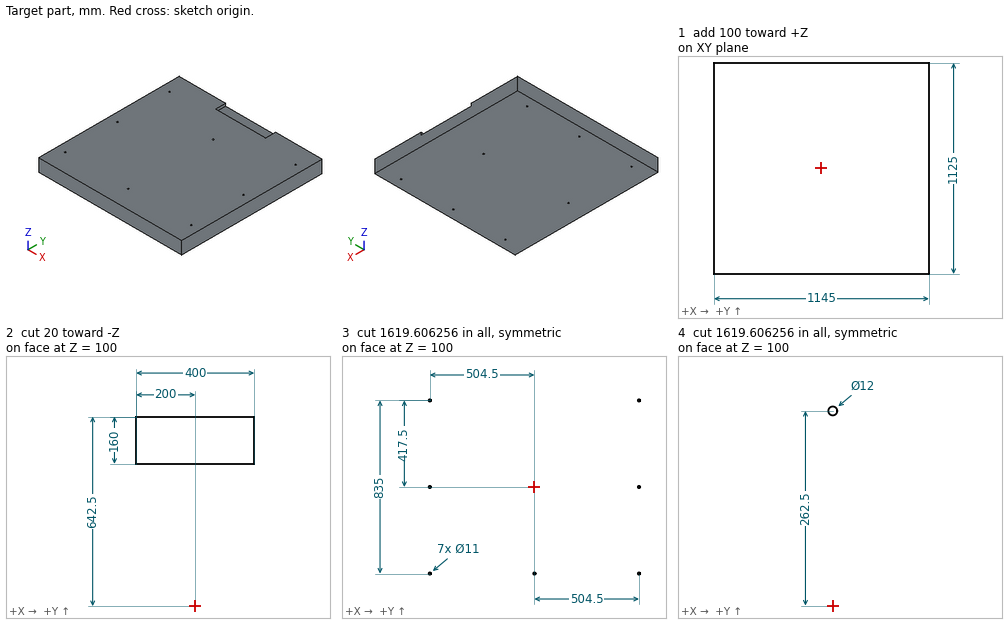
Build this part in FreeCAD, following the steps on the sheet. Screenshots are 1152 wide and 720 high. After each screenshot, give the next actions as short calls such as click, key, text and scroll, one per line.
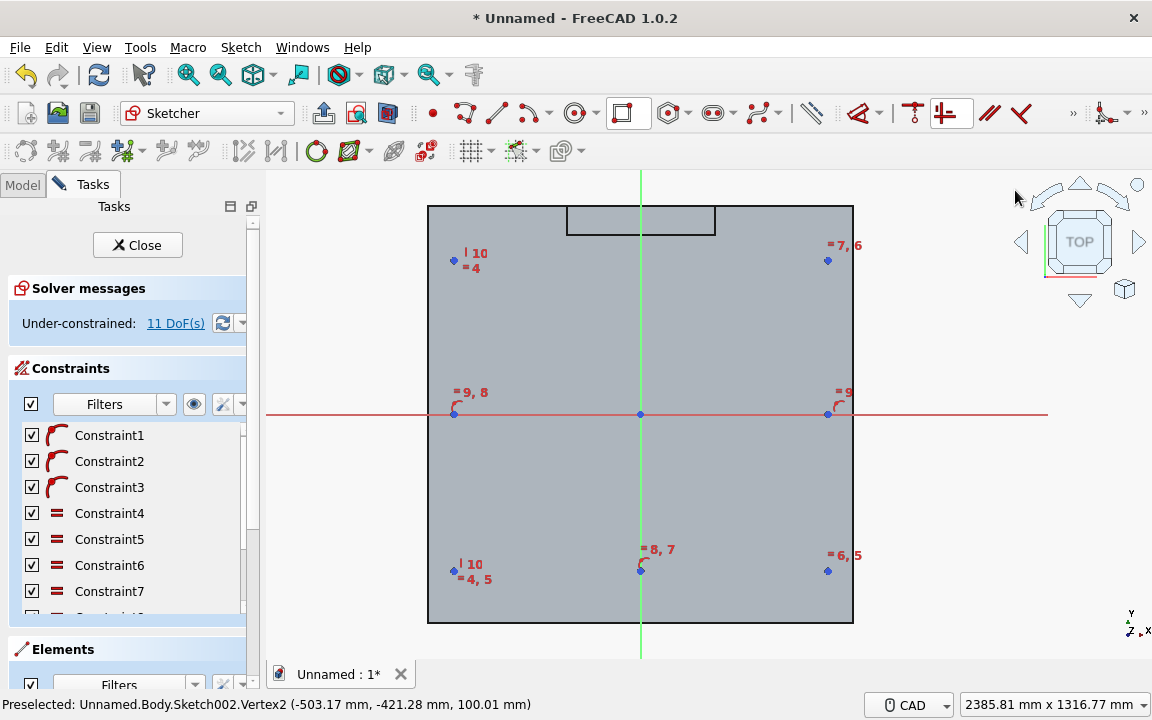
click(454, 571)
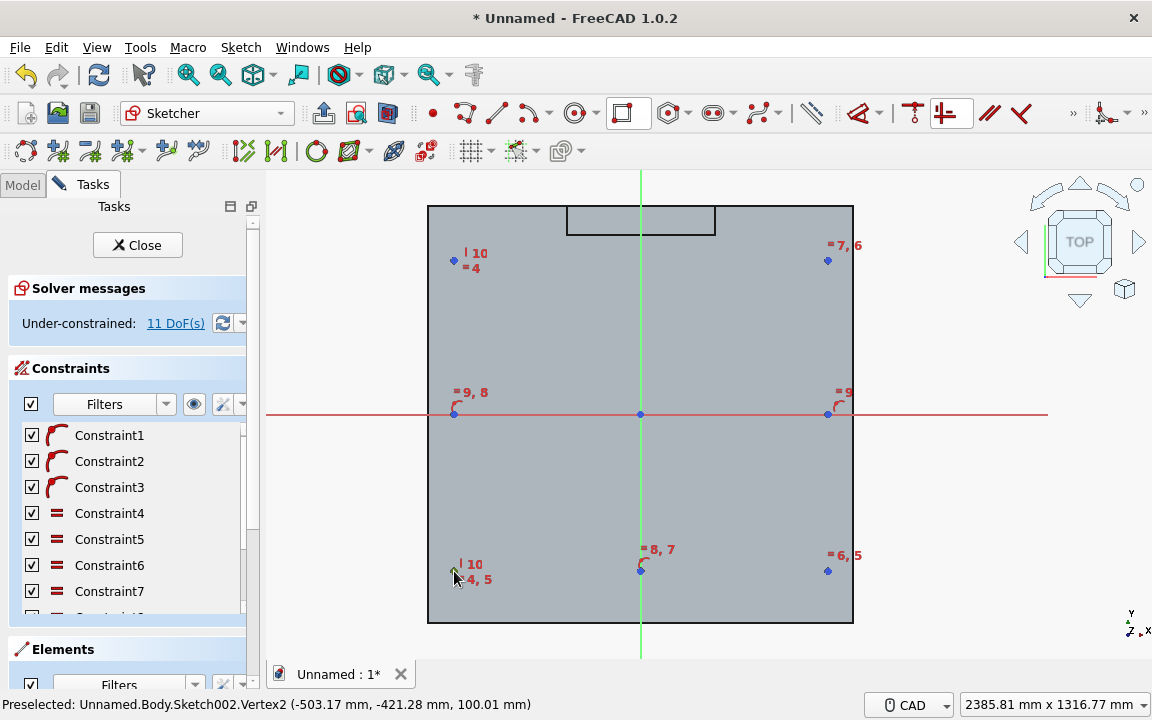
click(828, 571)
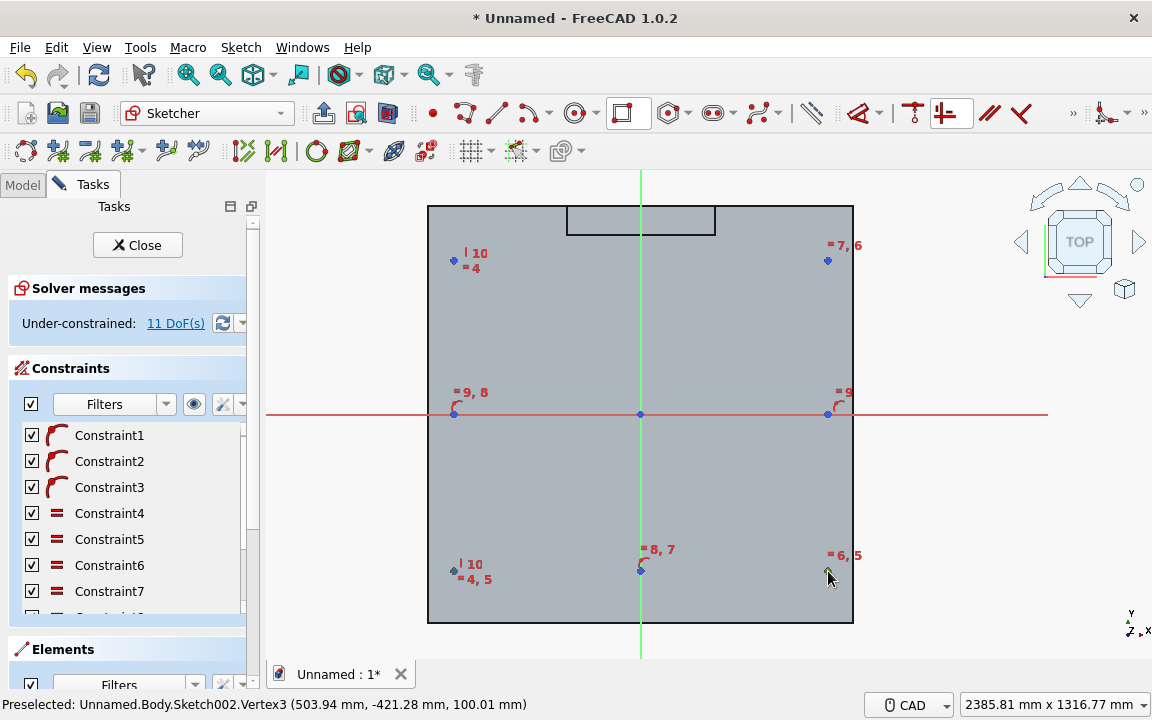
key(h)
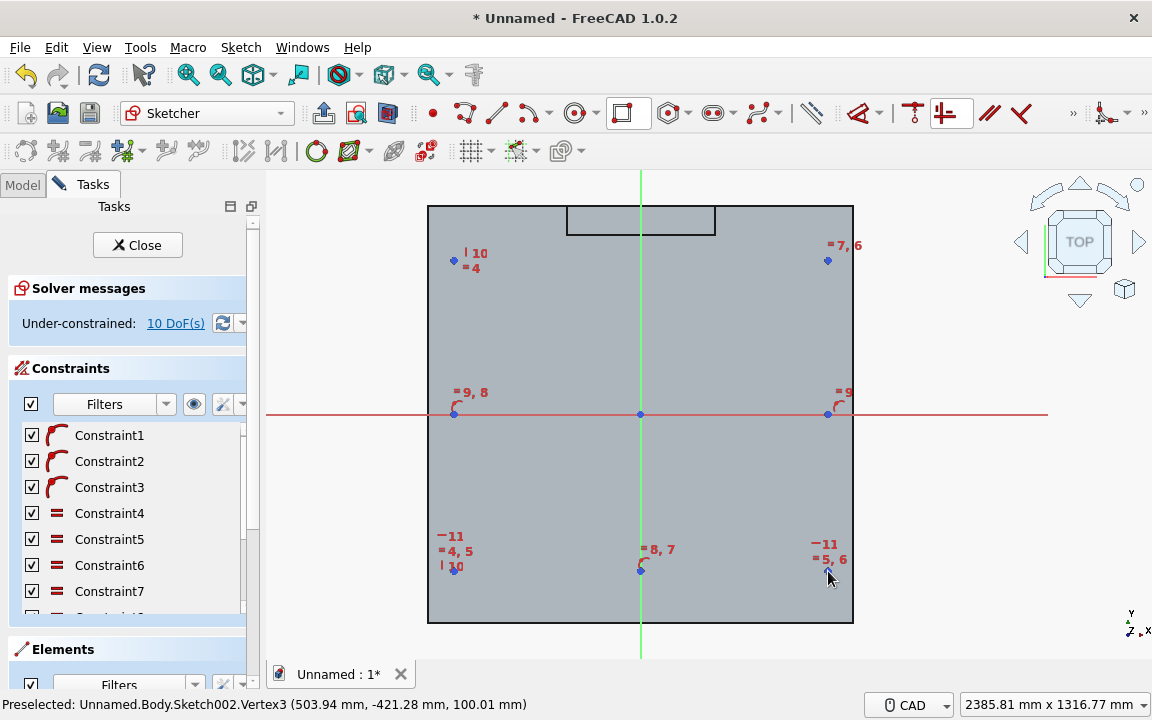
click(828, 571)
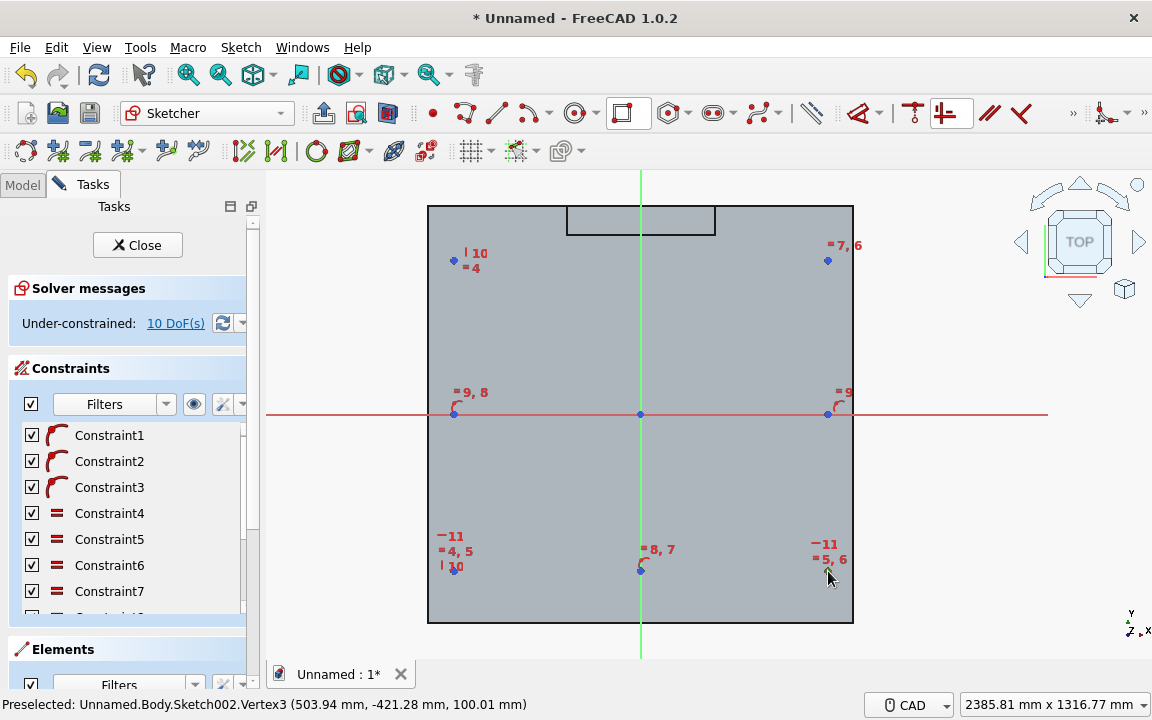
click(828, 261)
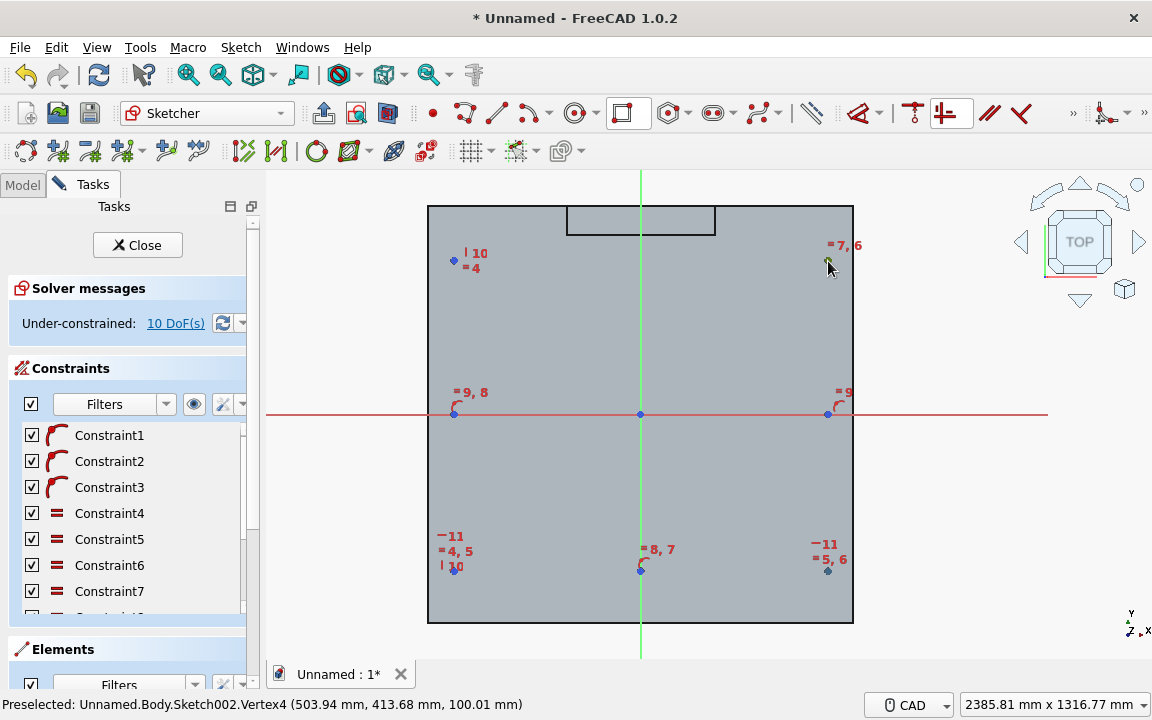
key(v)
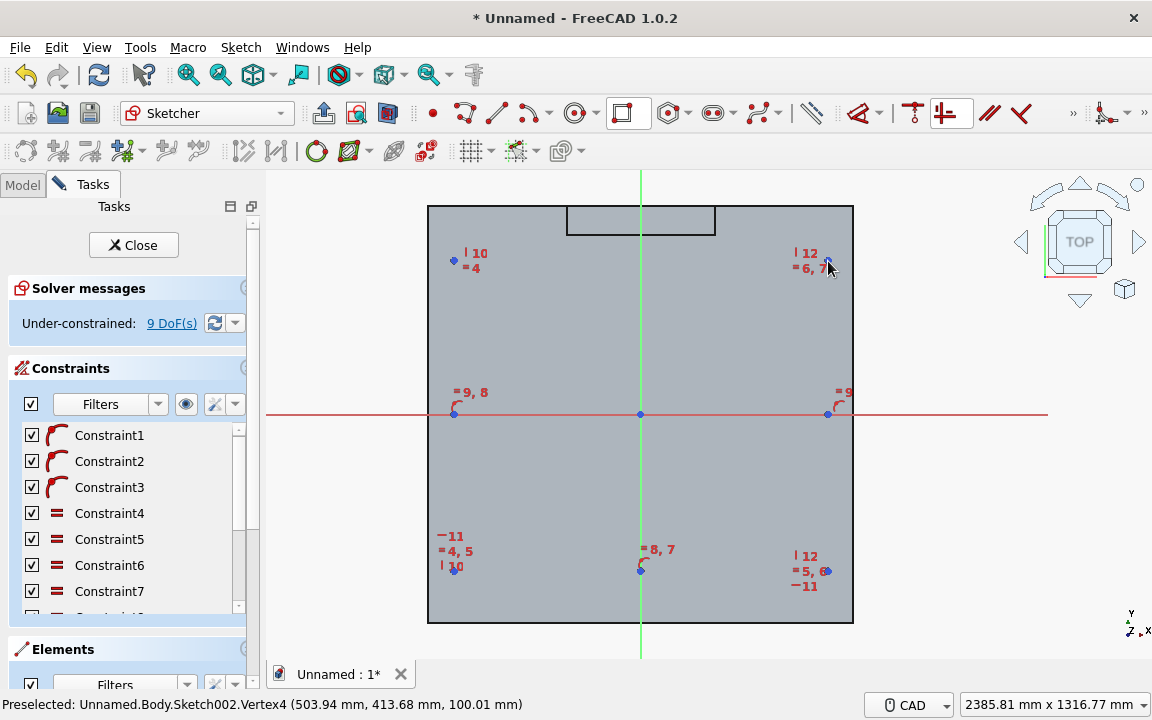
click(454, 261)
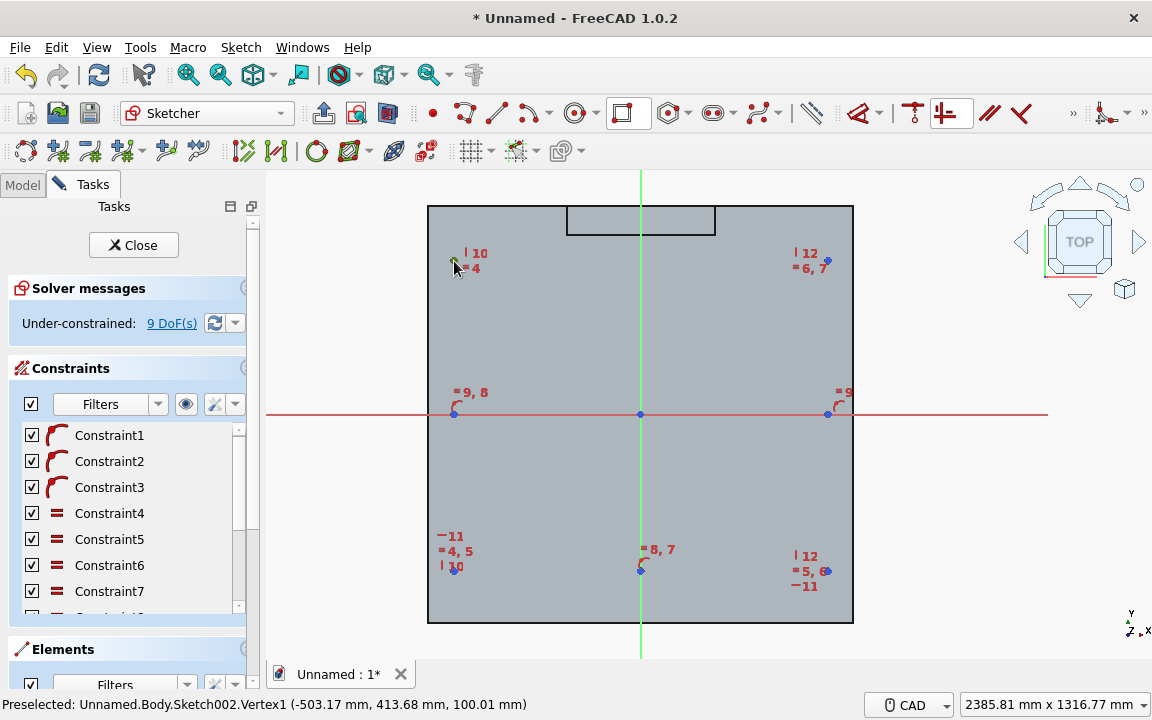
click(828, 261)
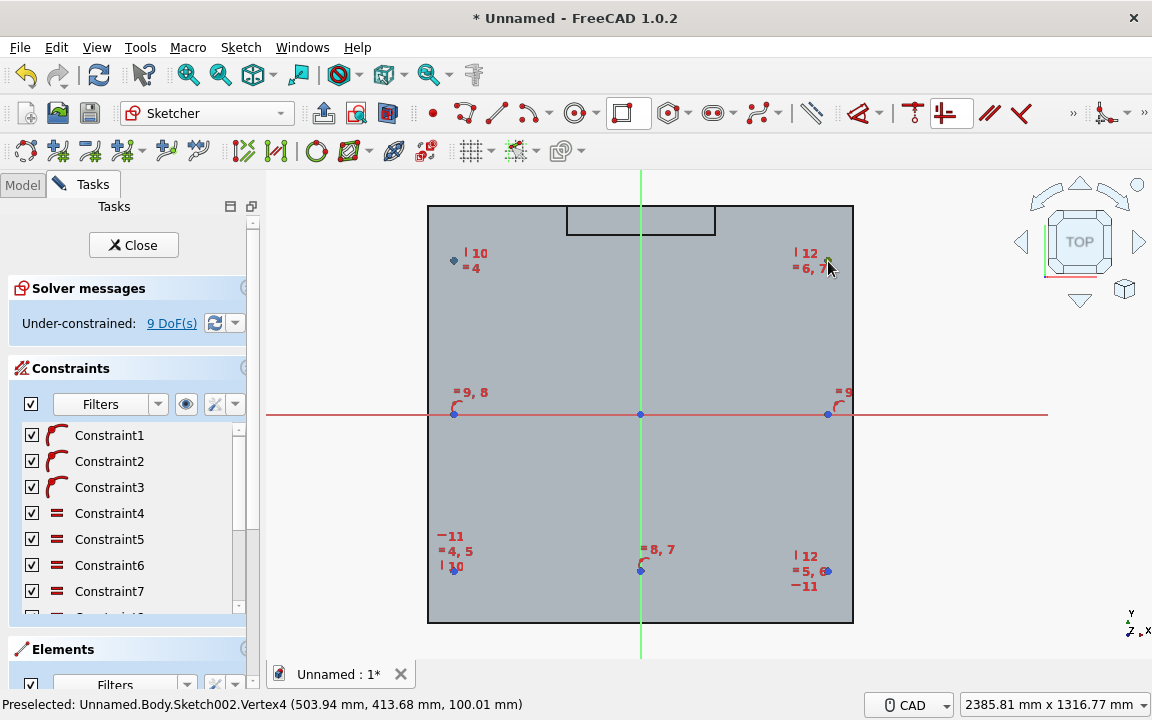
key(h)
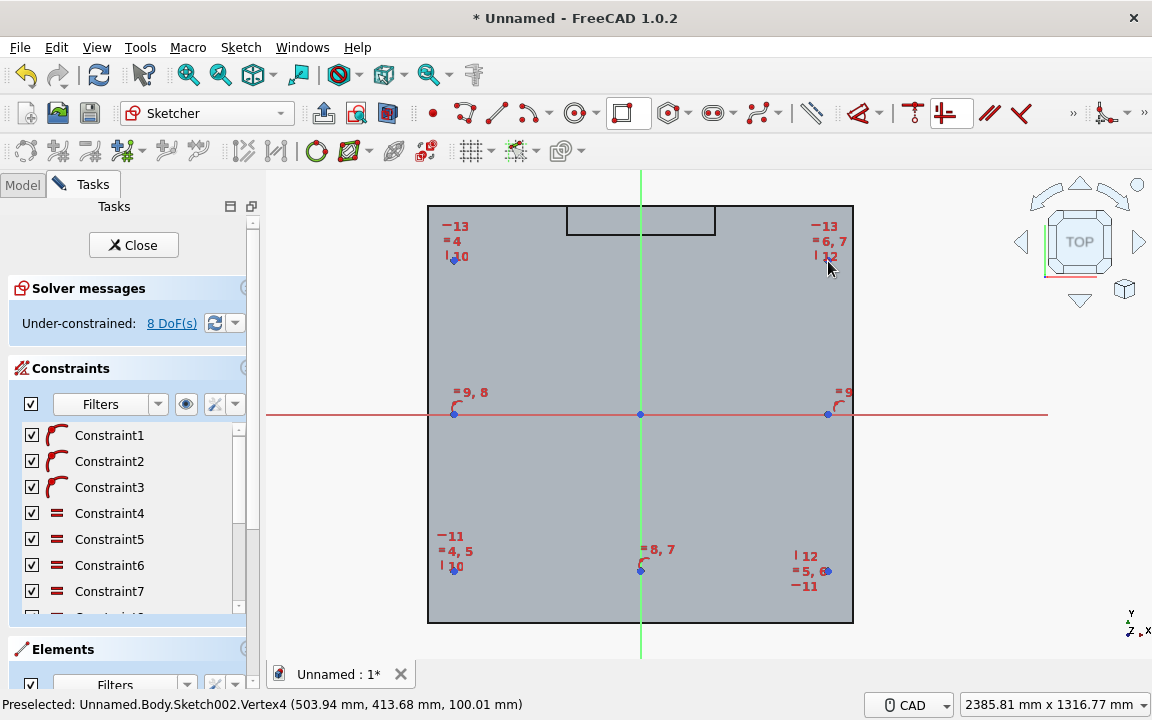
click(454, 571)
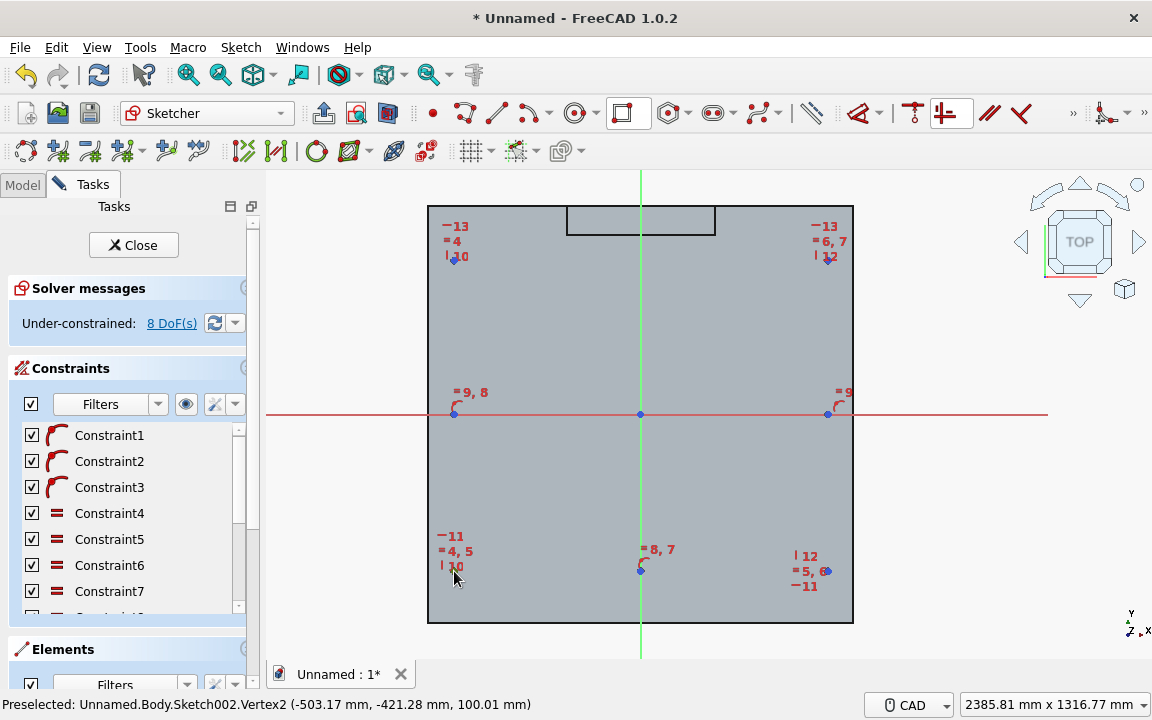
click(641, 571)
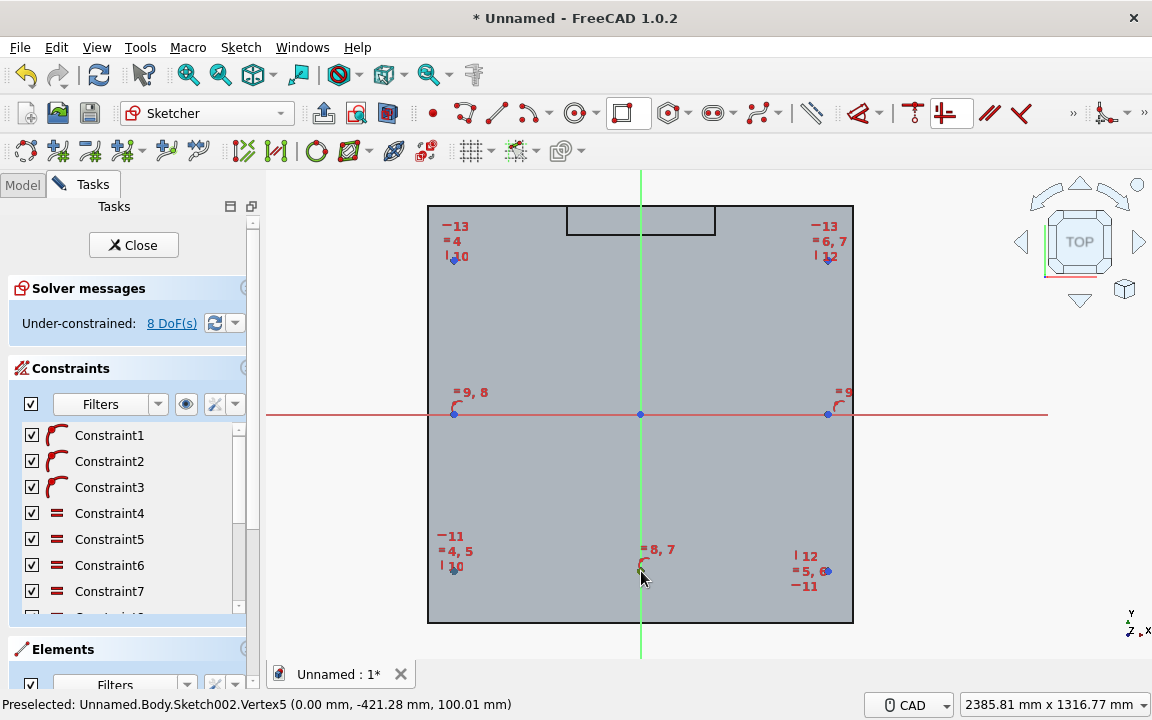
key(h)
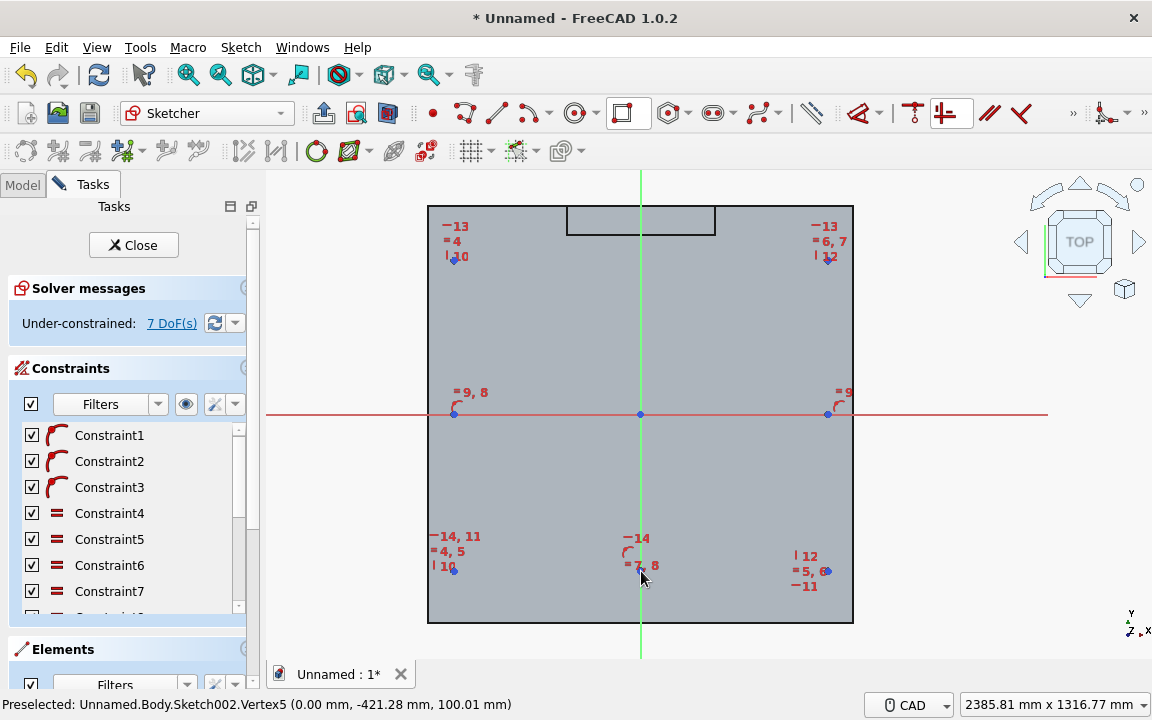
click(454, 261)